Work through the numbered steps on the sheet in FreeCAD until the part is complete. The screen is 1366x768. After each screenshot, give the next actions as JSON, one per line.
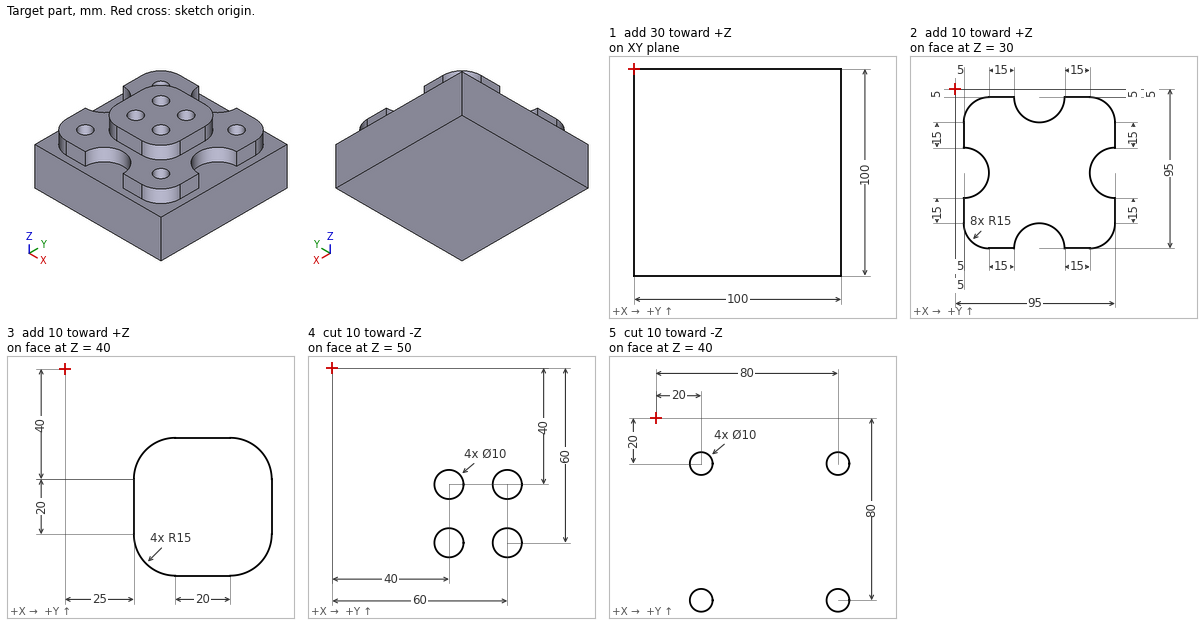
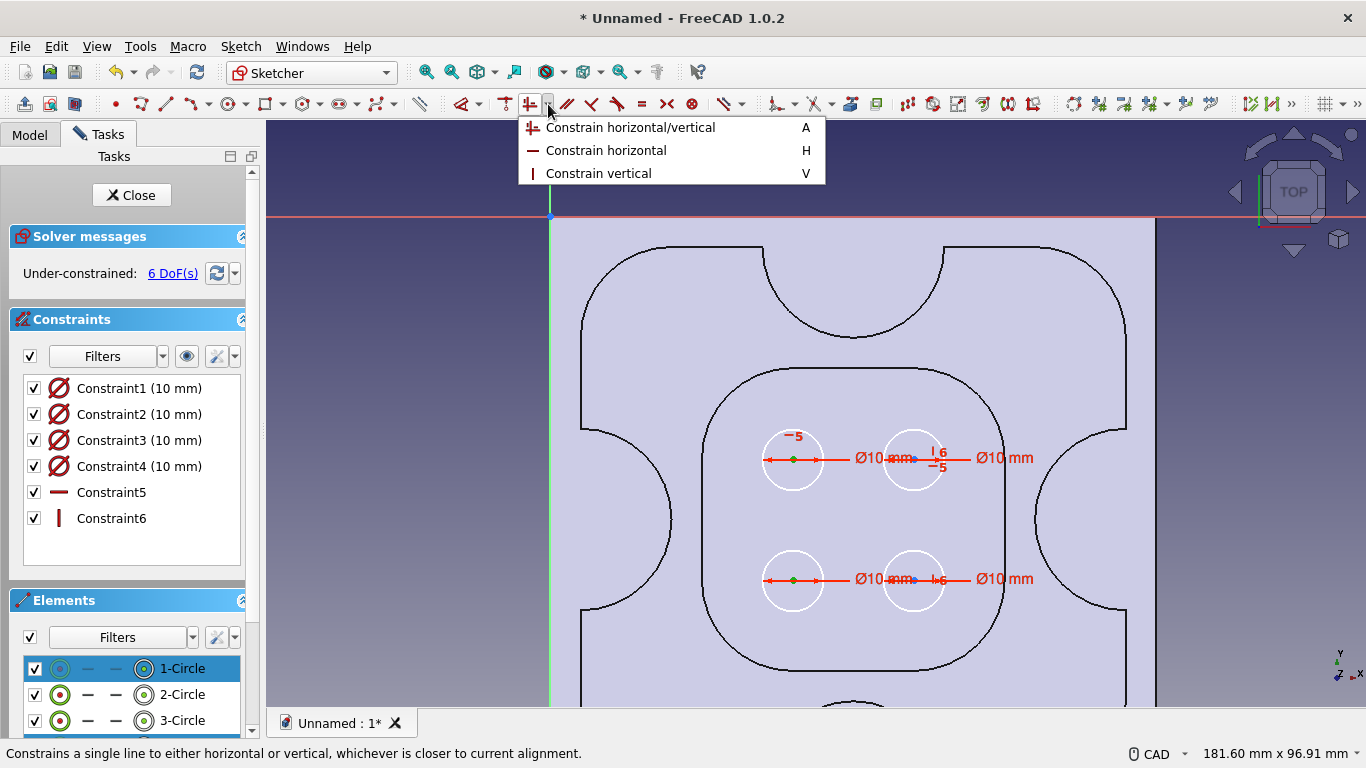
{"action": "left_click", "coordinate": [672, 174]}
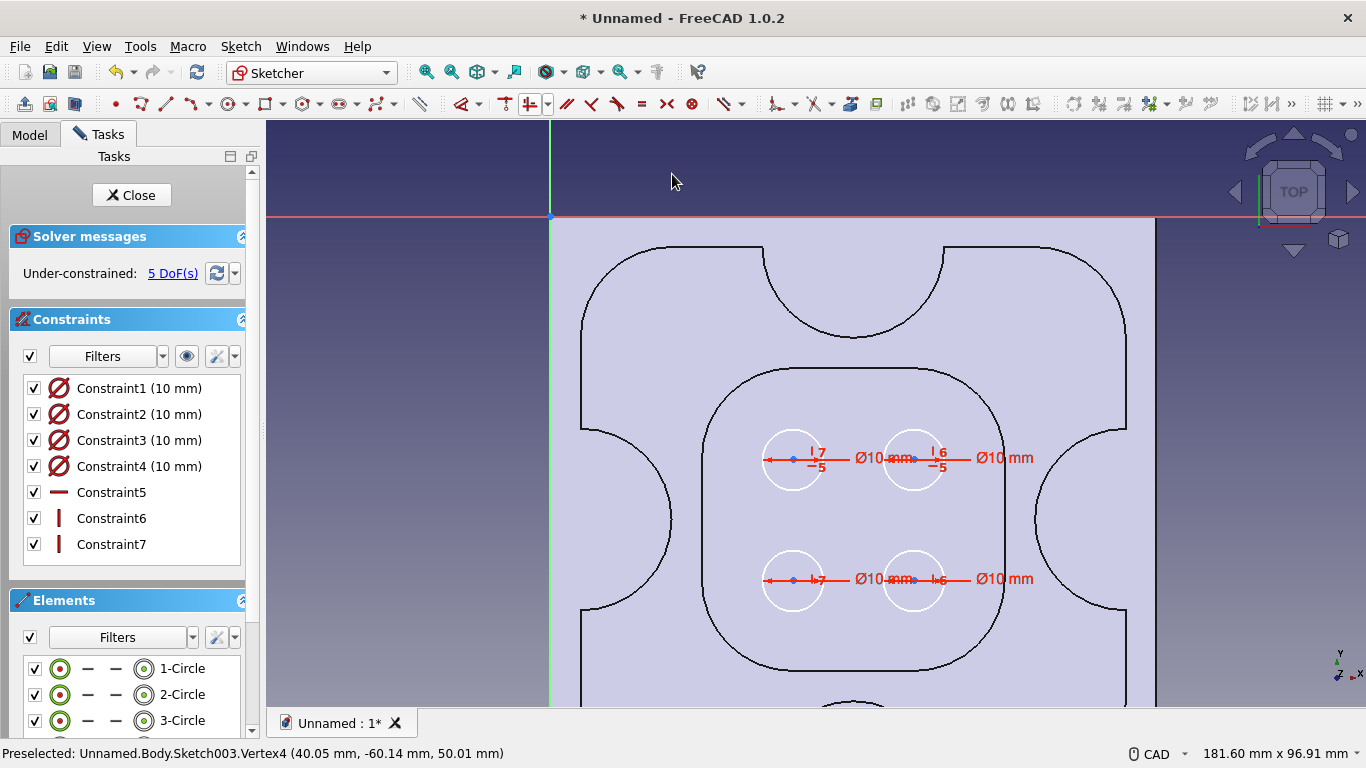
{"action": "left_click", "coordinate": [914, 581]}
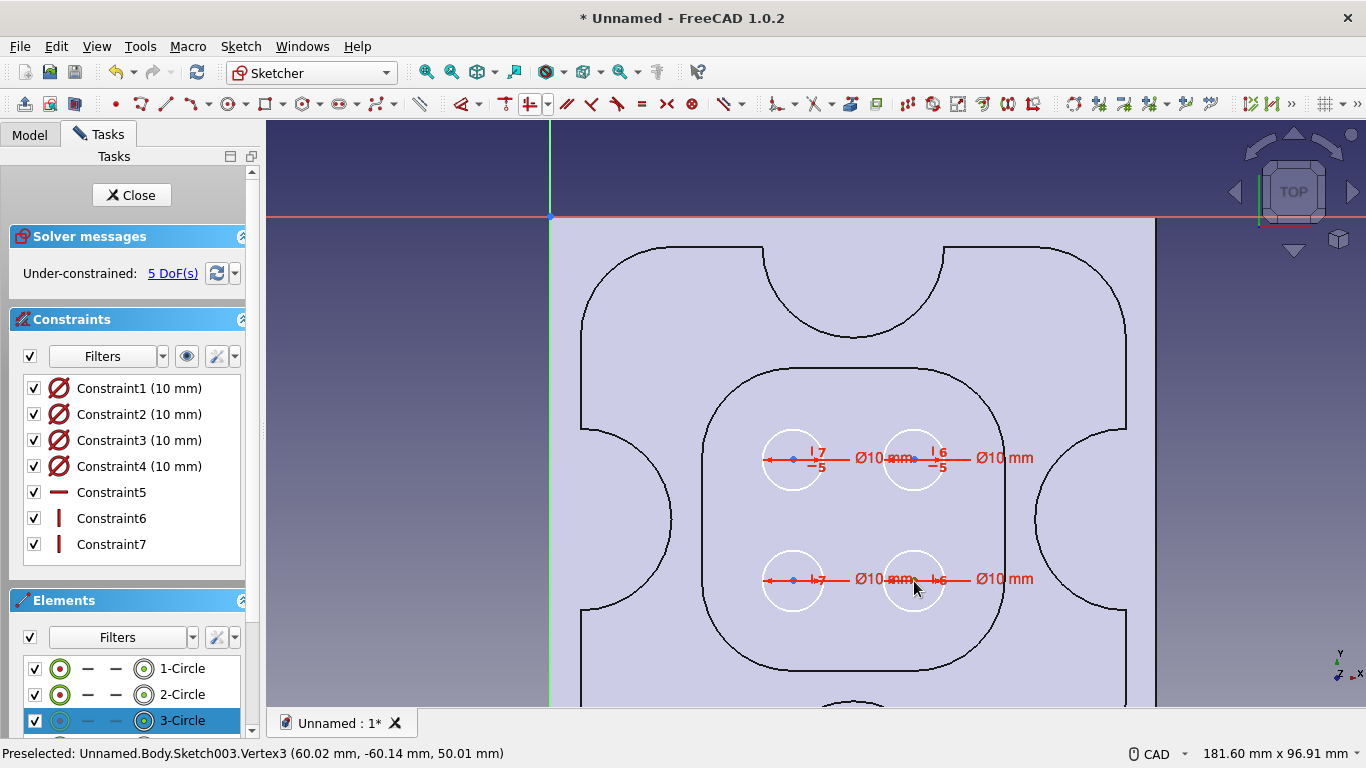
{"action": "left_click", "coordinate": [793, 581]}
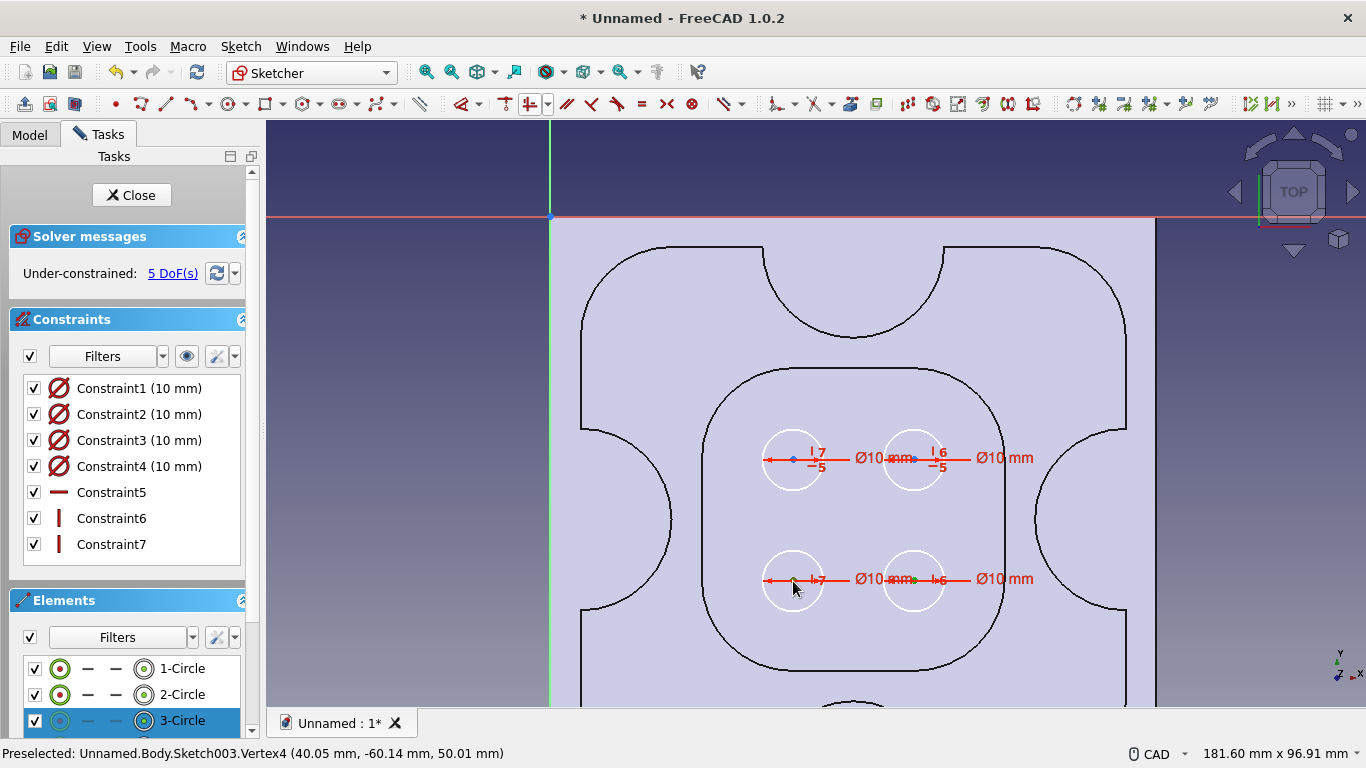
{"action": "key", "text": "h"}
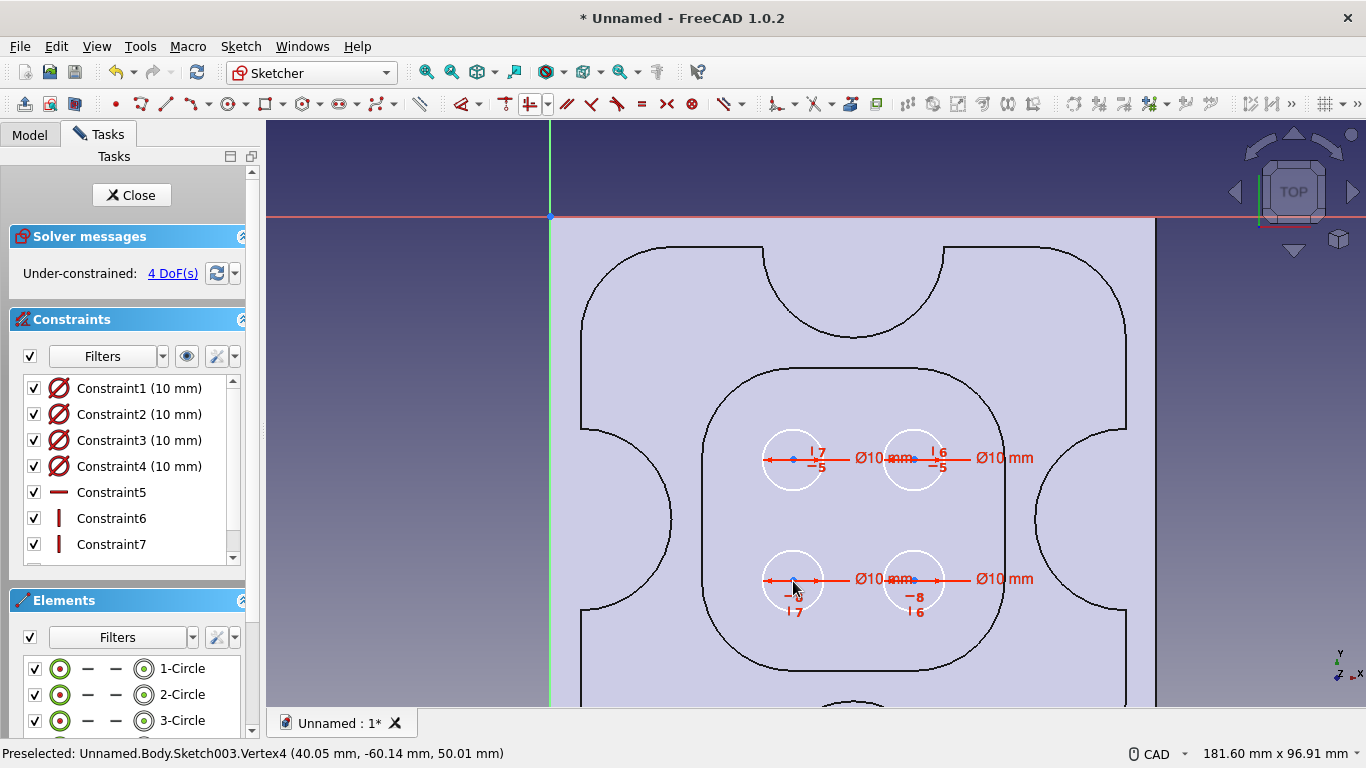
{"action": "left_click", "coordinate": [460, 104]}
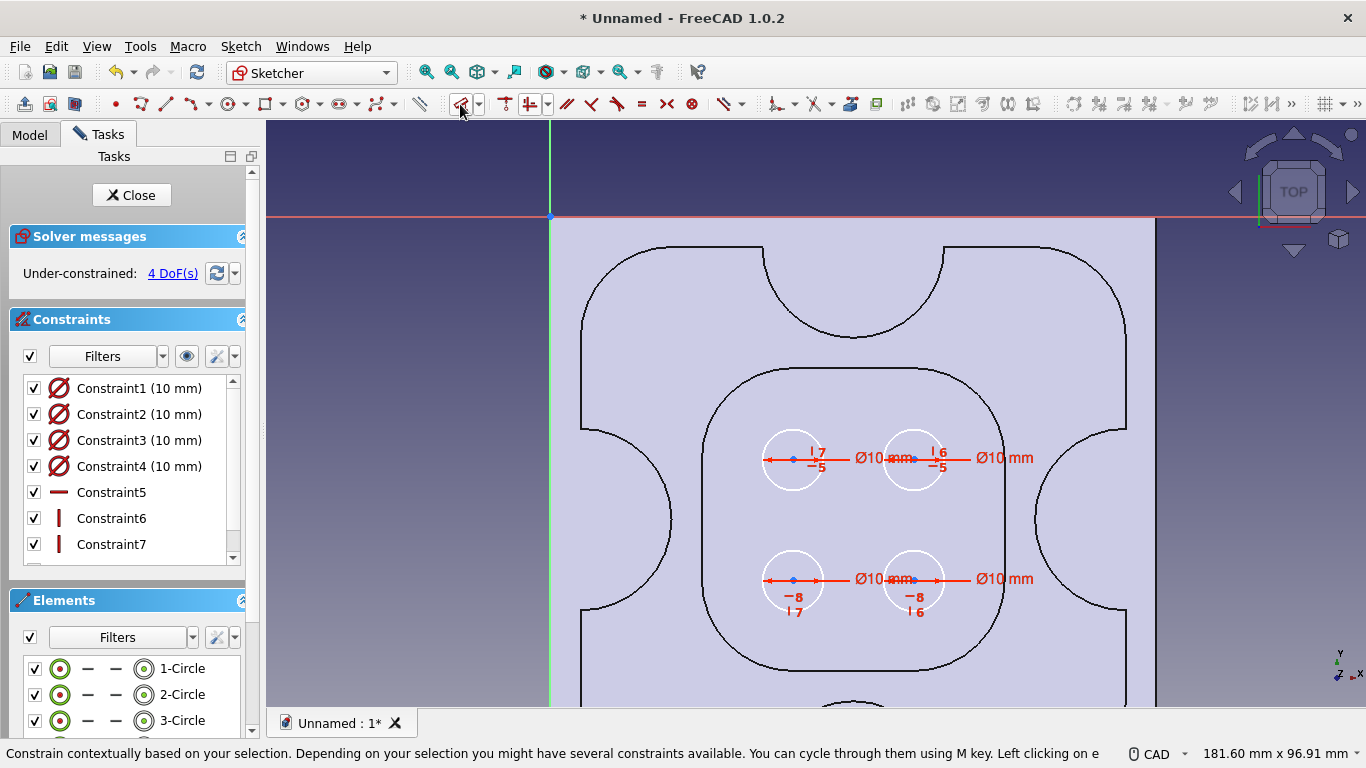
{"action": "left_click", "coordinate": [793, 460]}
{"action": "left_click", "coordinate": [672, 183]}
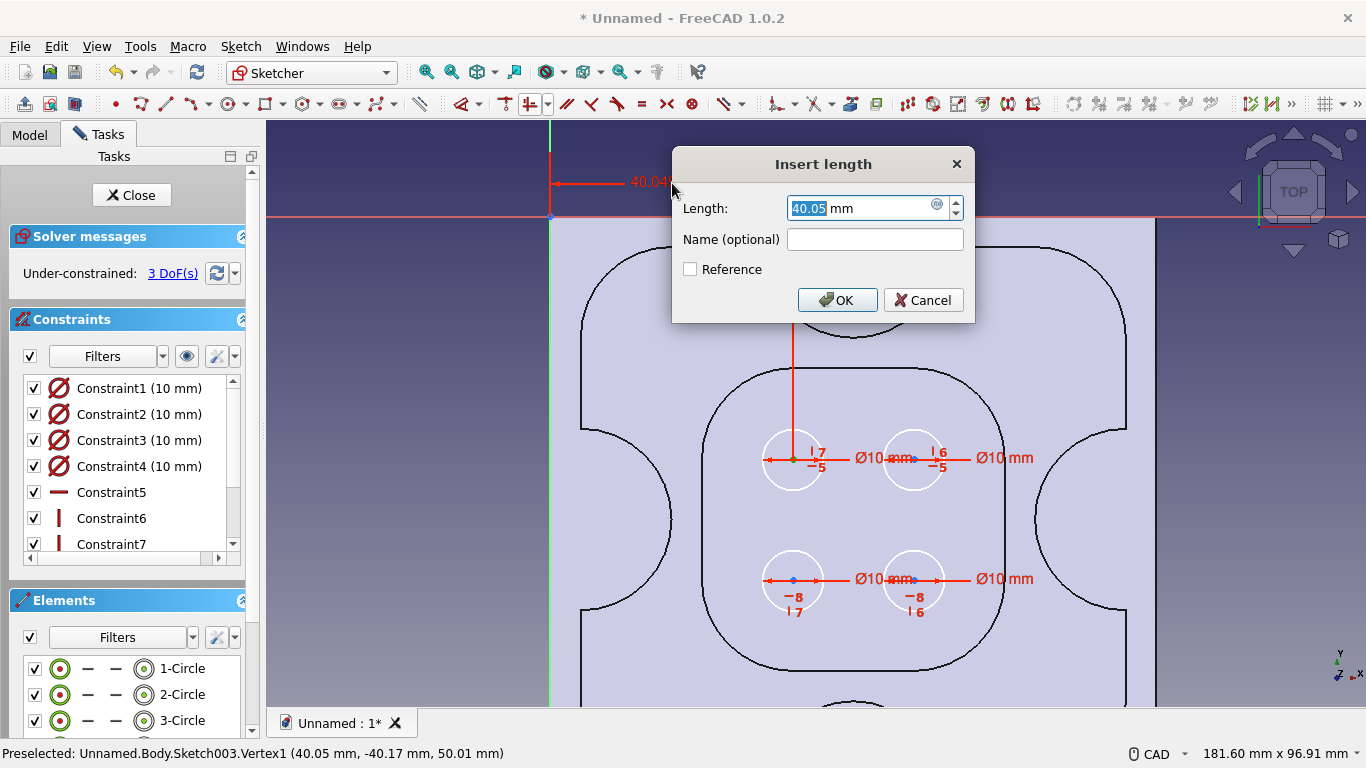
{"action": "type", "text": "40"}
{"action": "key", "text": "Return"}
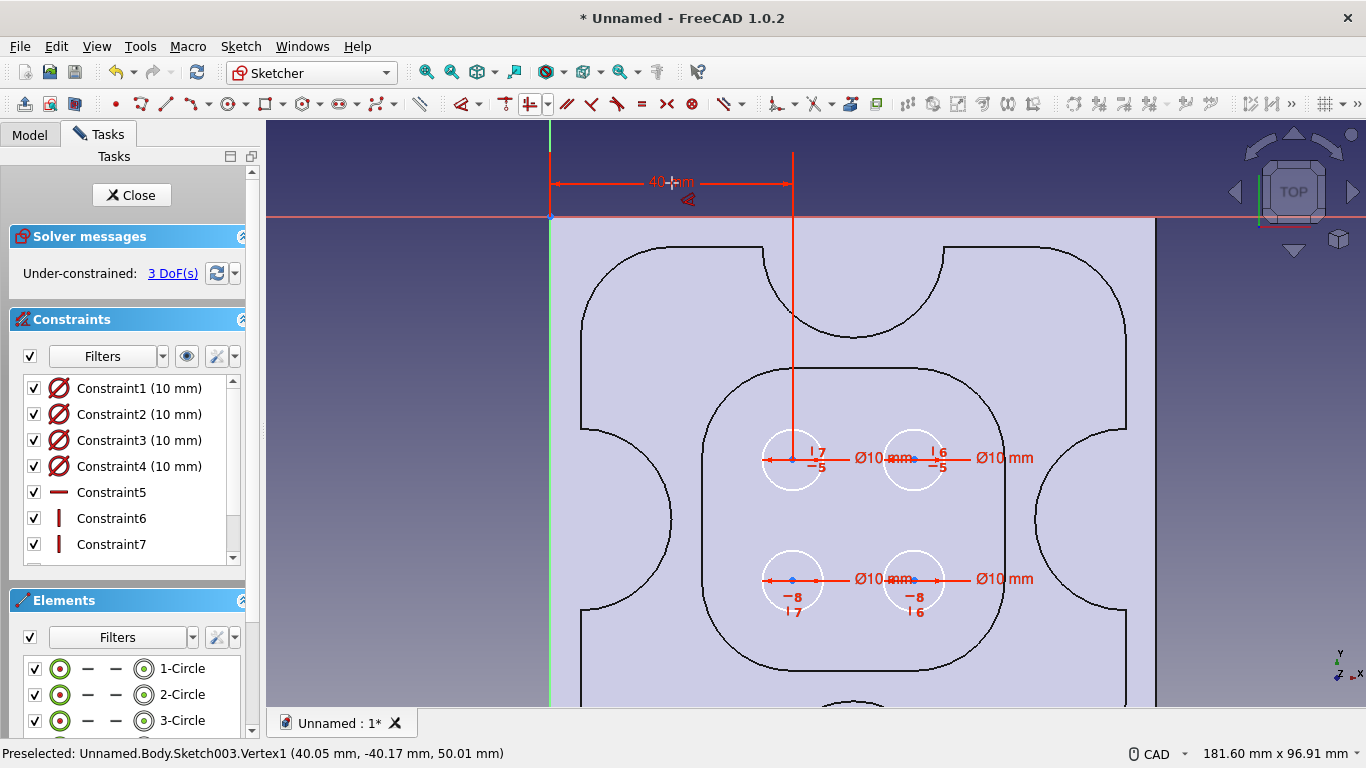
{"action": "left_click", "coordinate": [793, 460]}
{"action": "left_click", "coordinate": [516, 338]}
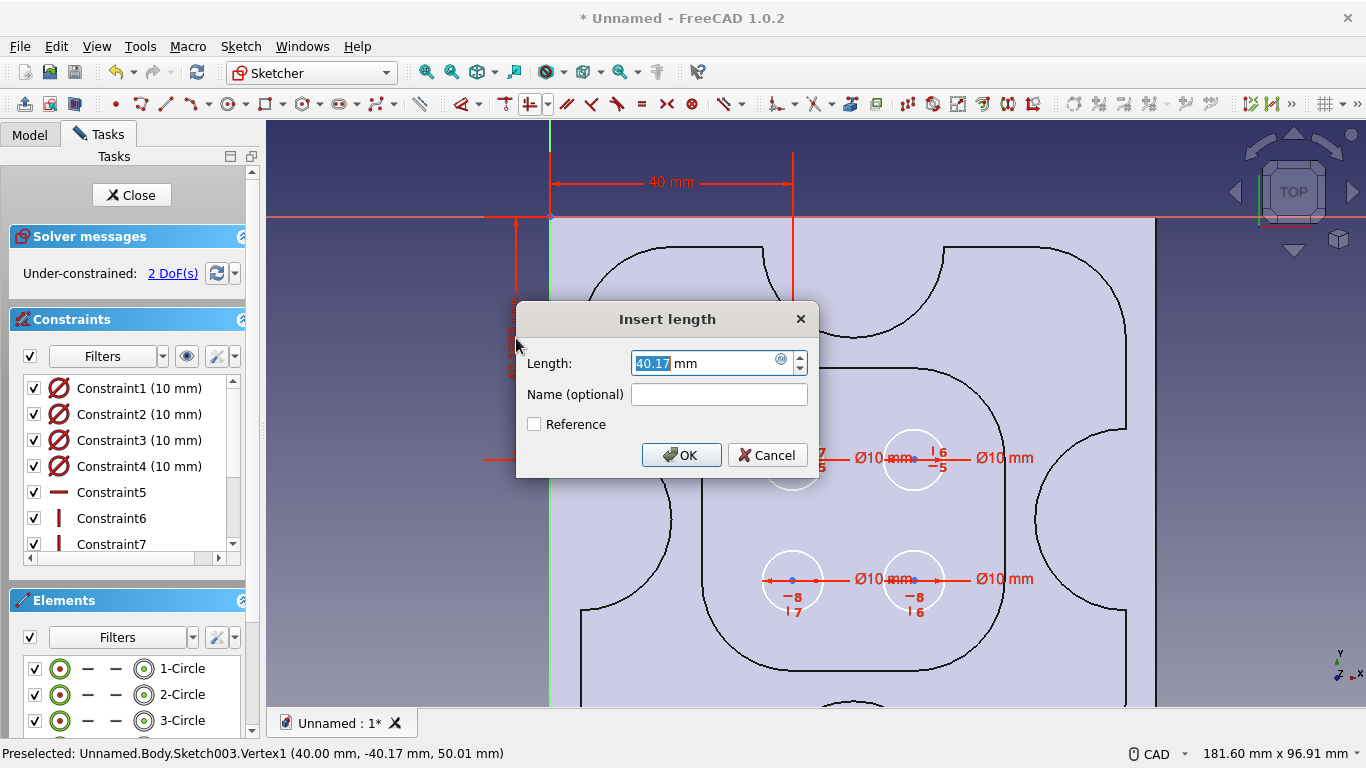
{"action": "type", "text": "40"}
{"action": "key", "text": "Return"}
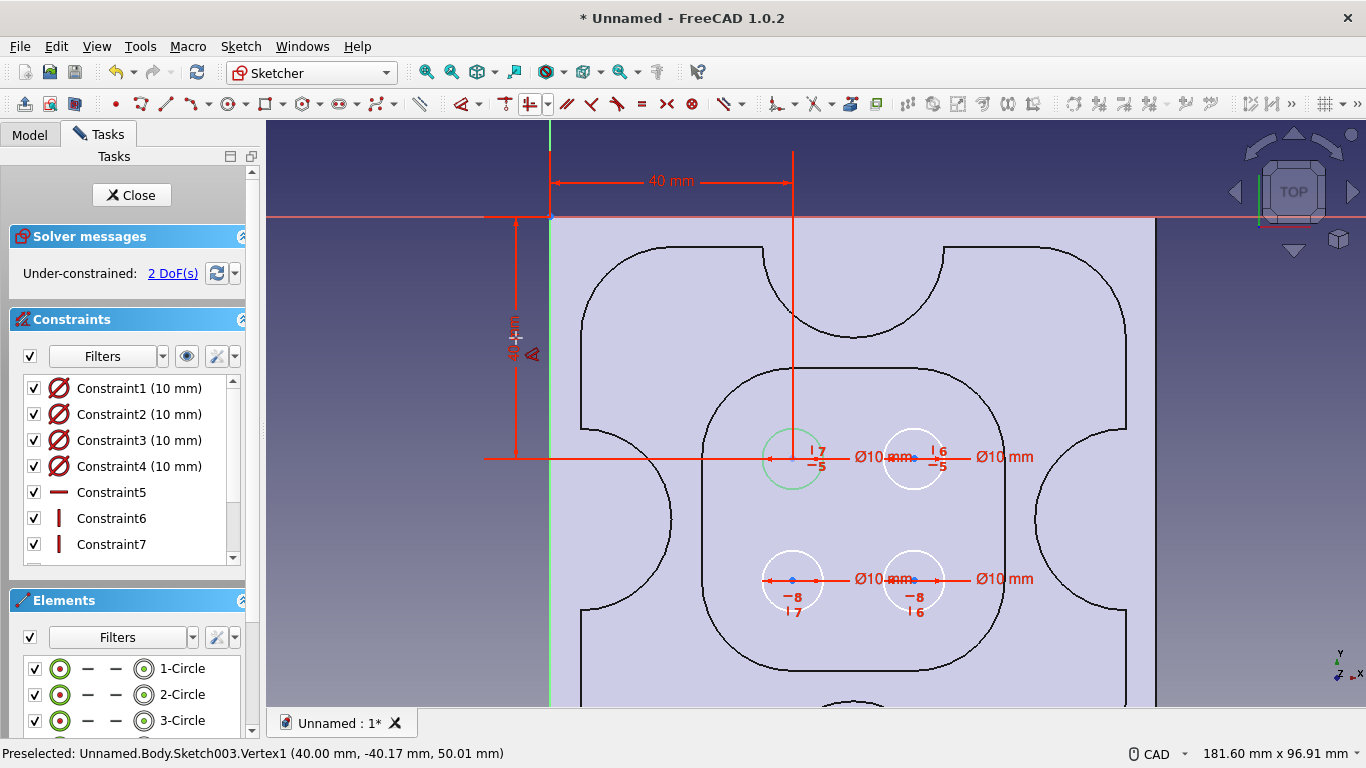
{"action": "left_click", "coordinate": [914, 459]}
{"action": "left_click", "coordinate": [816, 183]}